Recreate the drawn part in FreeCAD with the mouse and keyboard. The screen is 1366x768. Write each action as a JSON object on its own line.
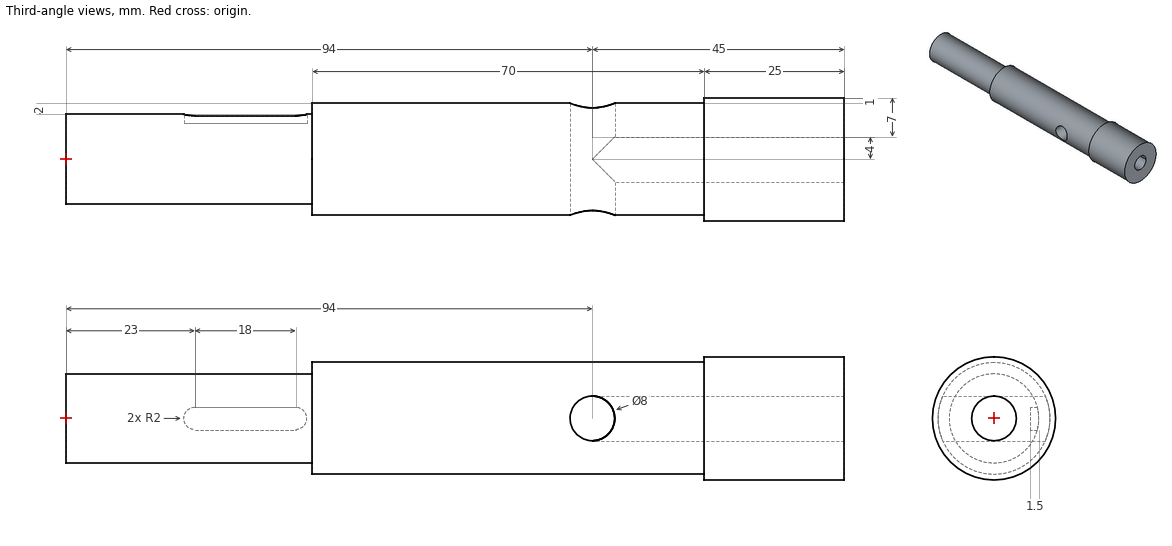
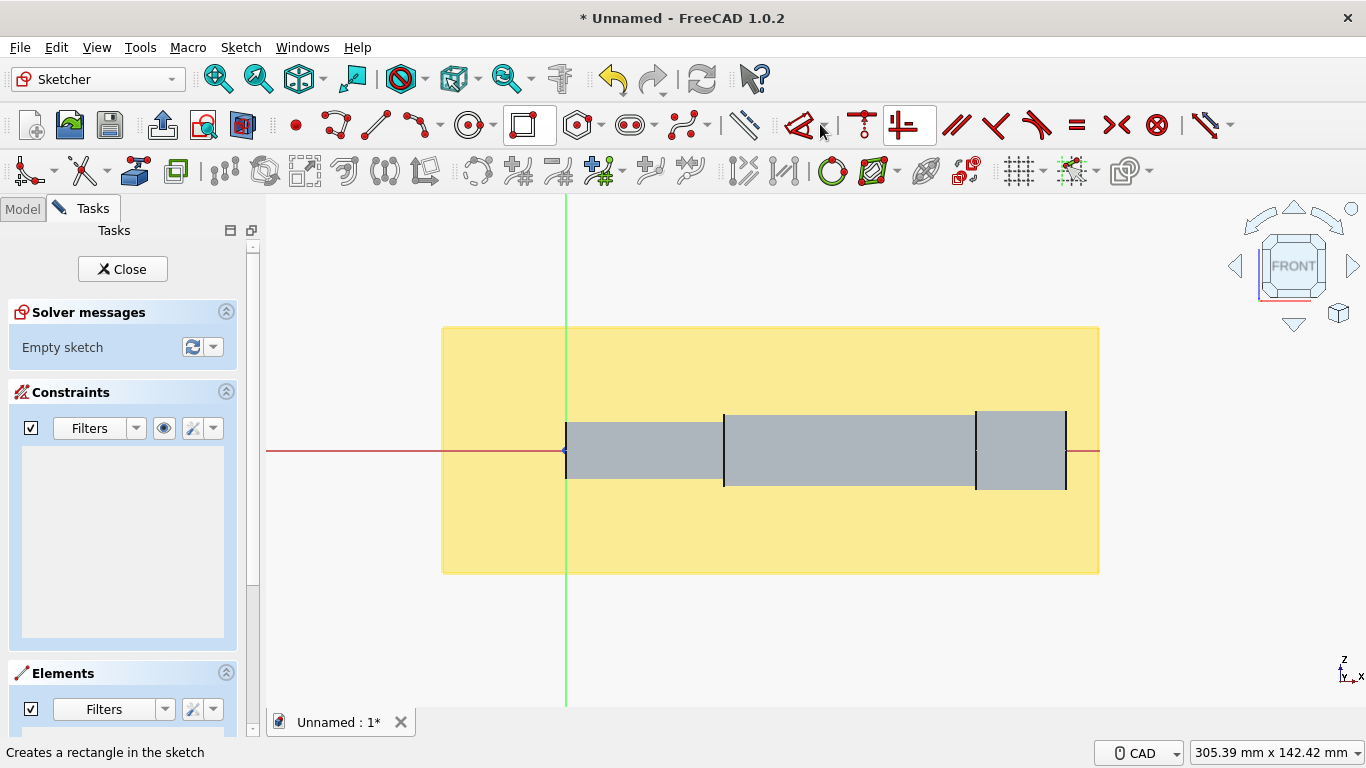
{"action": "key", "text": "q s"}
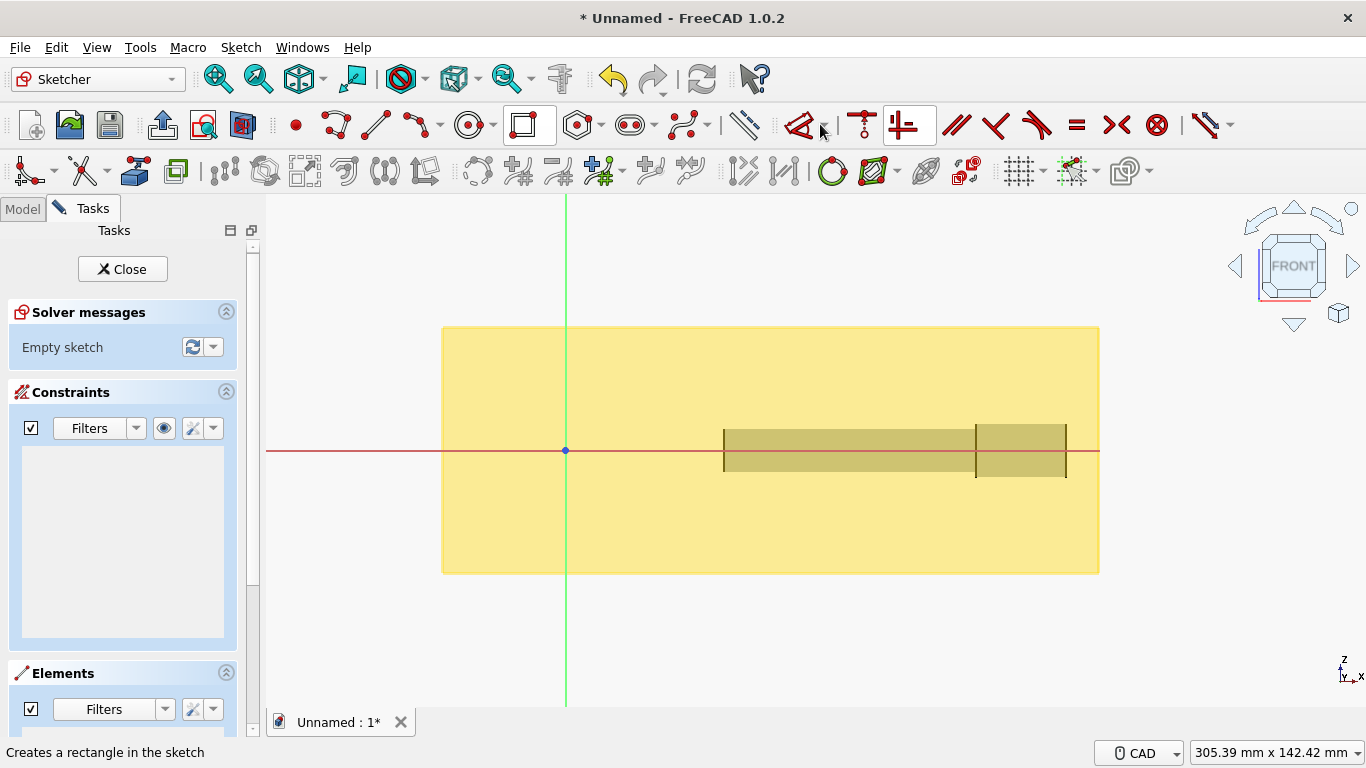
{"action": "scroll", "coordinate": [609, 450], "scroll_direction": "up", "scroll_amount": 7}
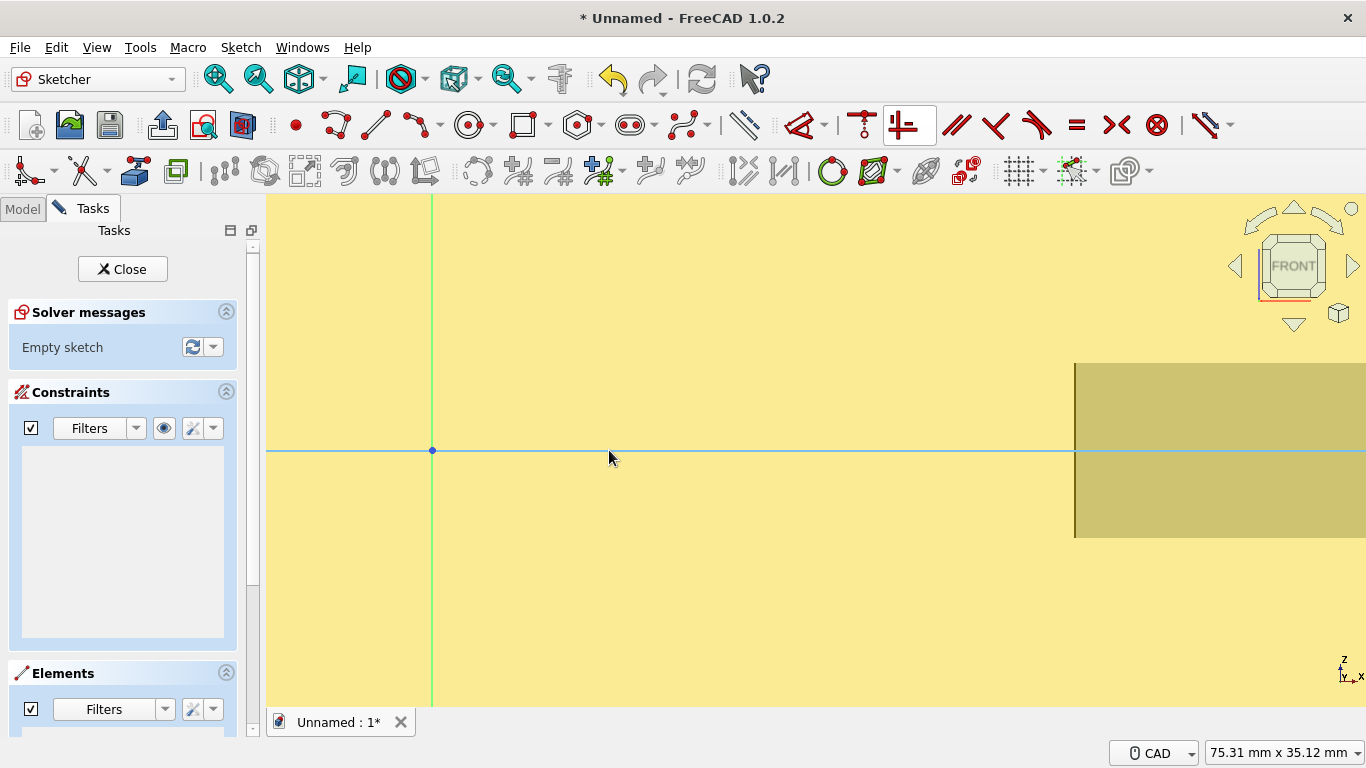
{"action": "left_click", "coordinate": [630, 126]}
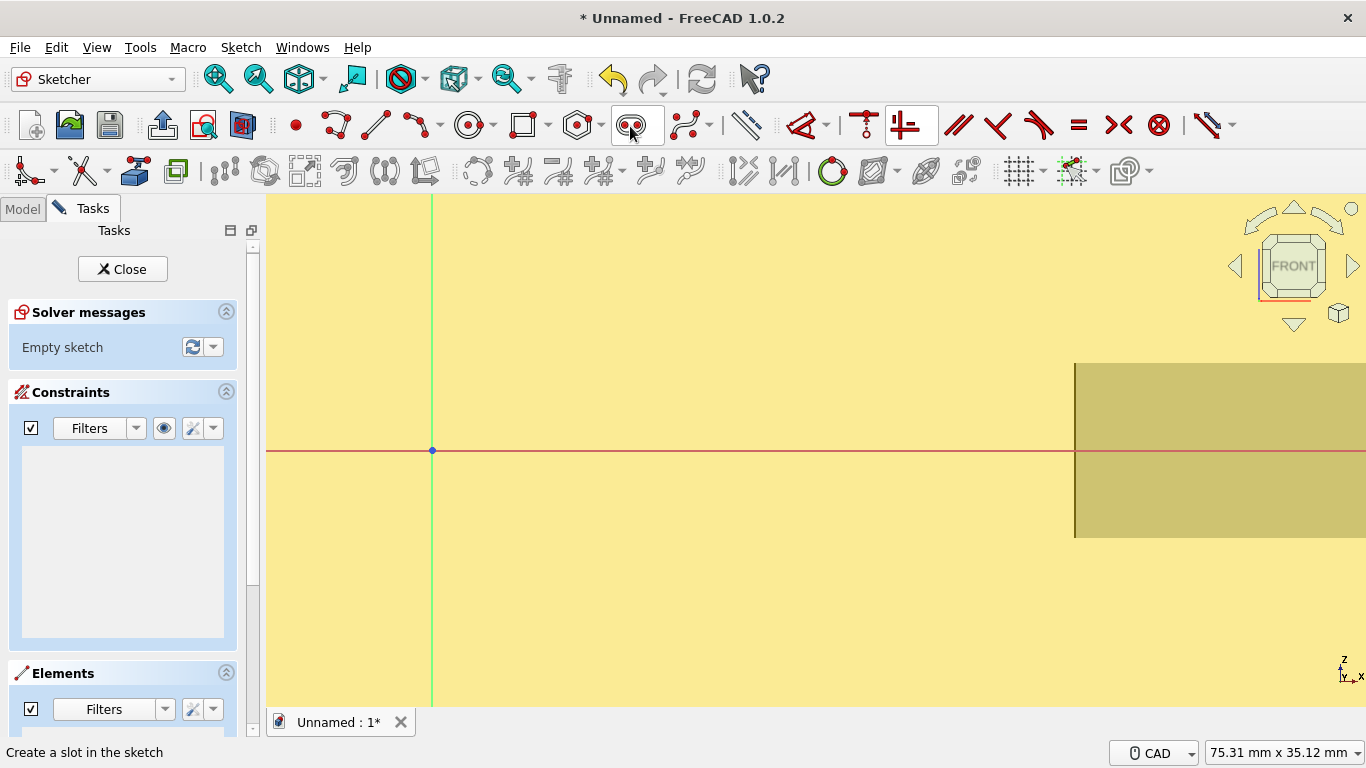
{"action": "left_click", "coordinate": [768, 450]}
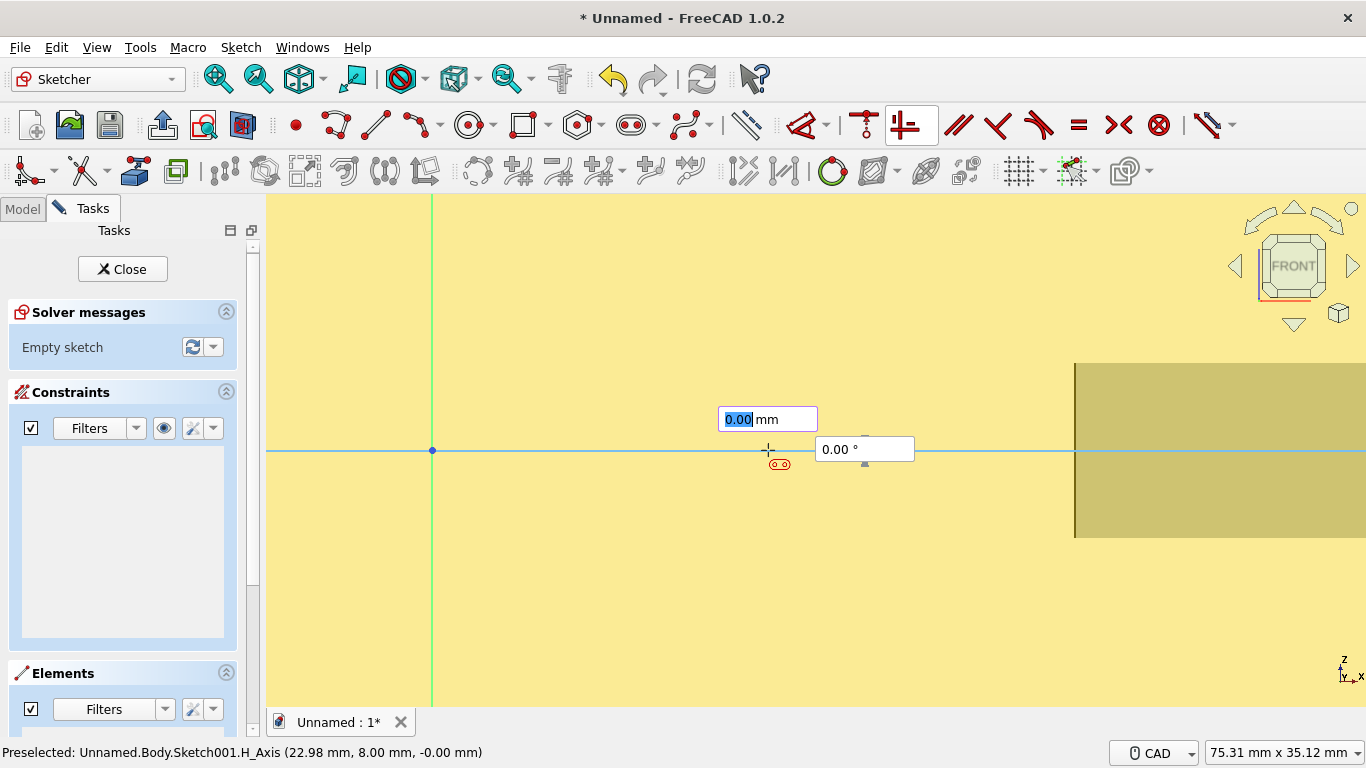
{"action": "left_click", "coordinate": [1031, 442]}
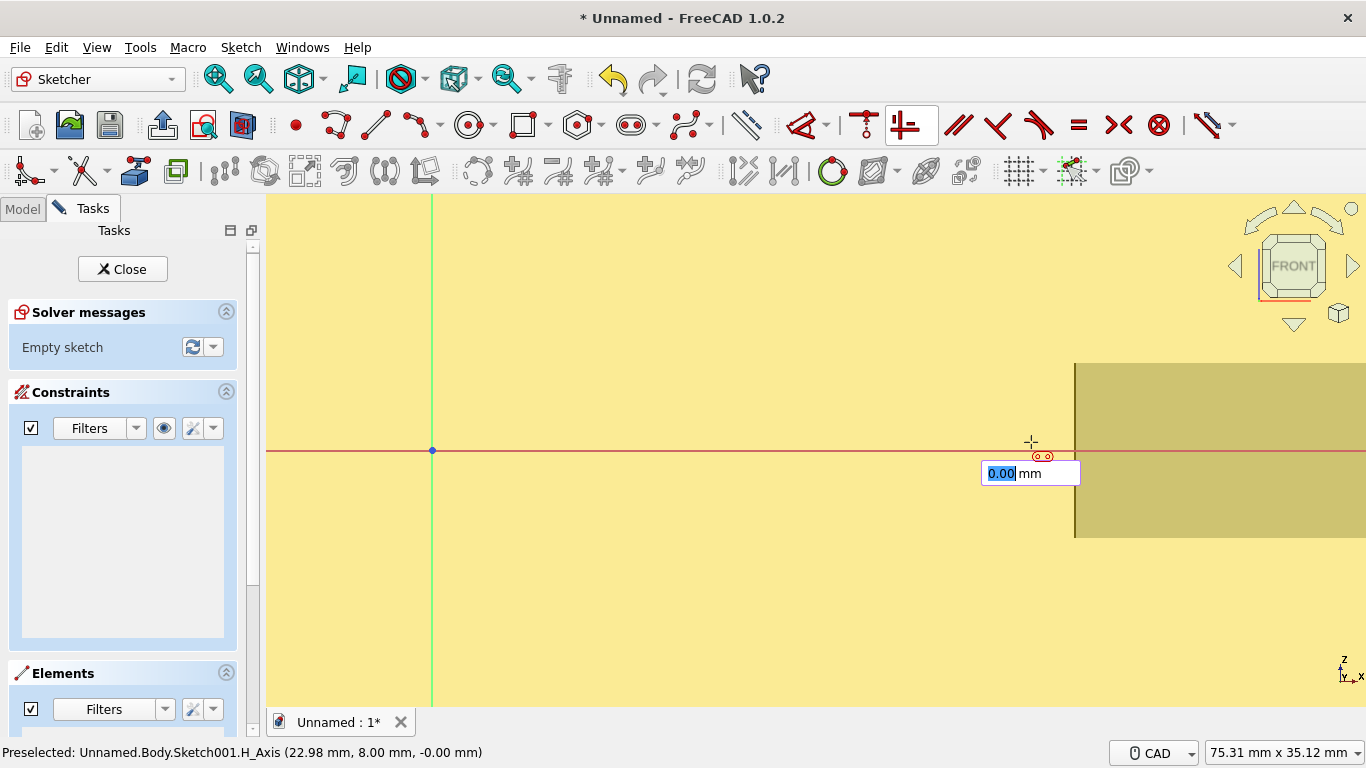
{"action": "left_click", "coordinate": [900, 480]}
{"action": "key", "text": "Escape"}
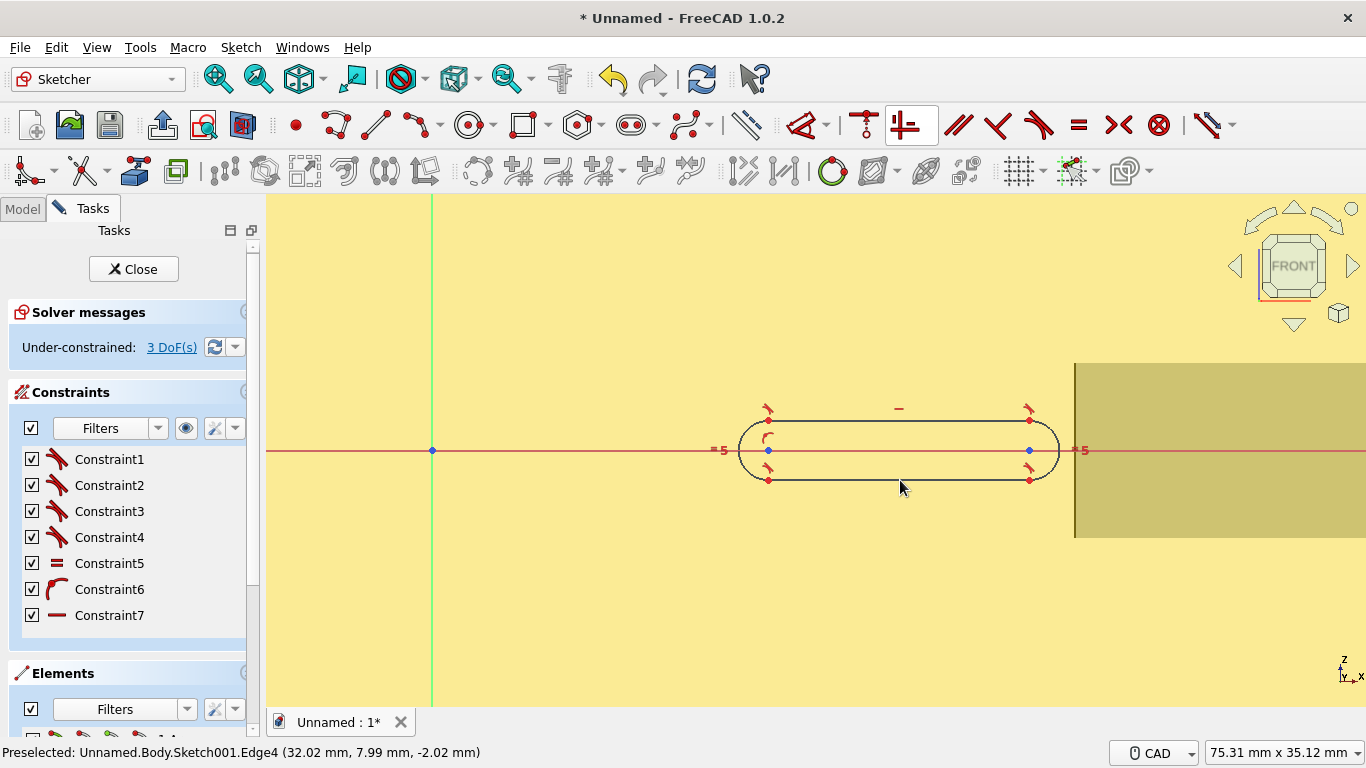
{"action": "key", "text": "d"}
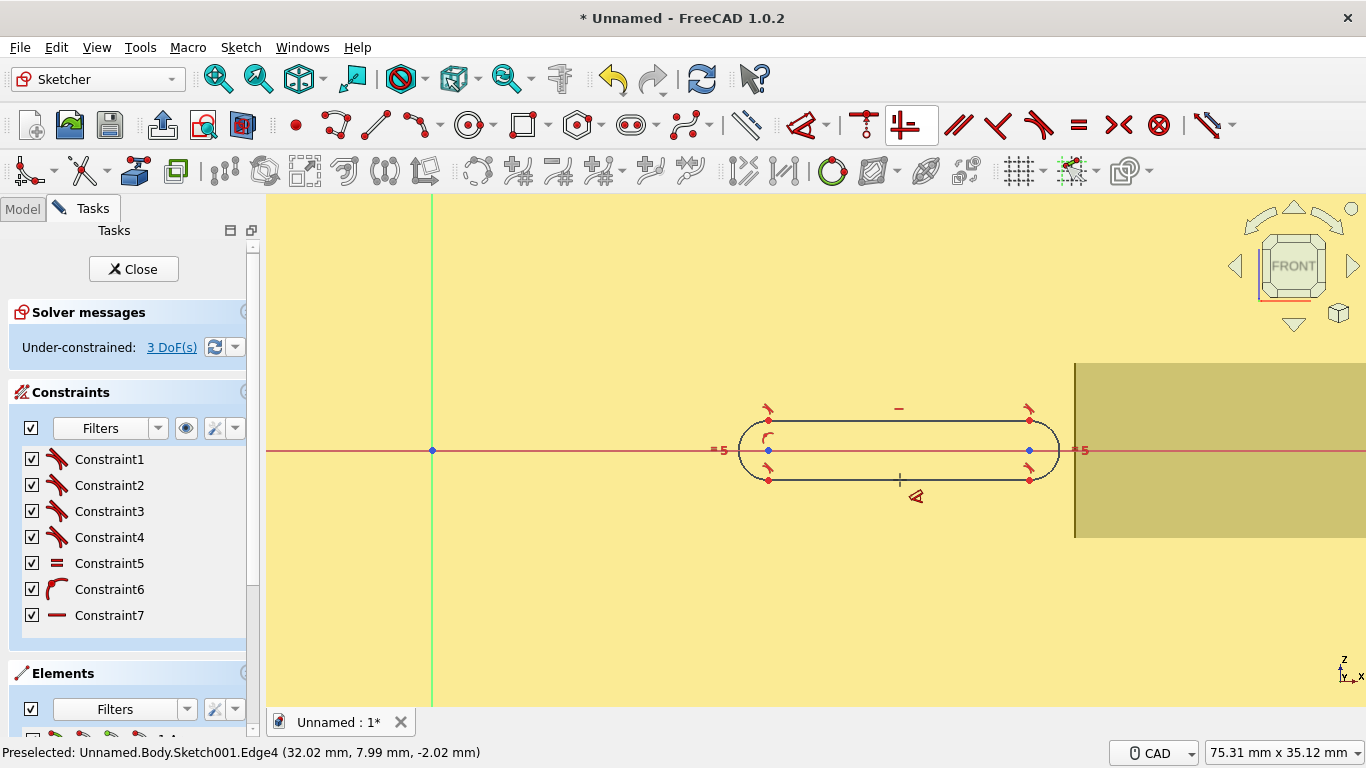
{"action": "scroll", "coordinate": [745, 433], "scroll_direction": "up", "scroll_amount": 2}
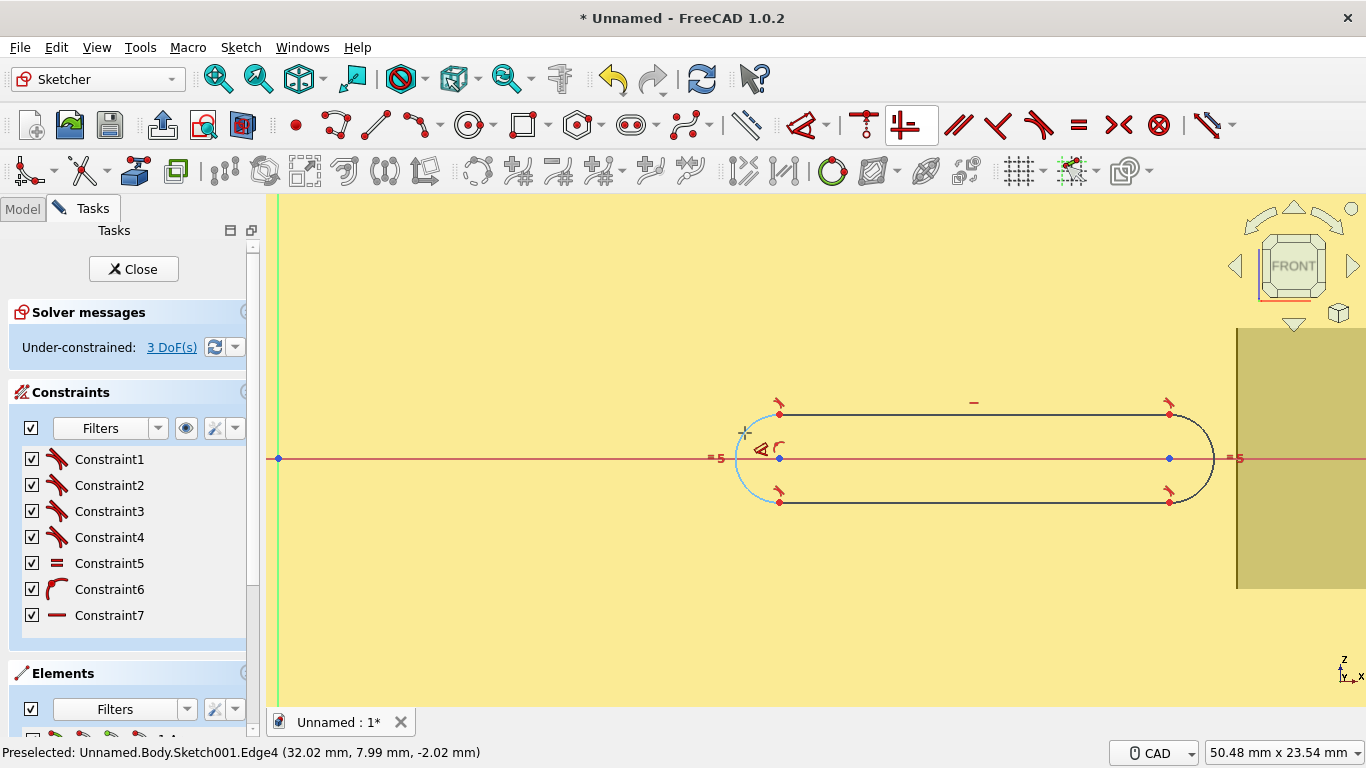
{"action": "left_click", "coordinate": [744, 433]}
{"action": "left_click", "coordinate": [718, 414]}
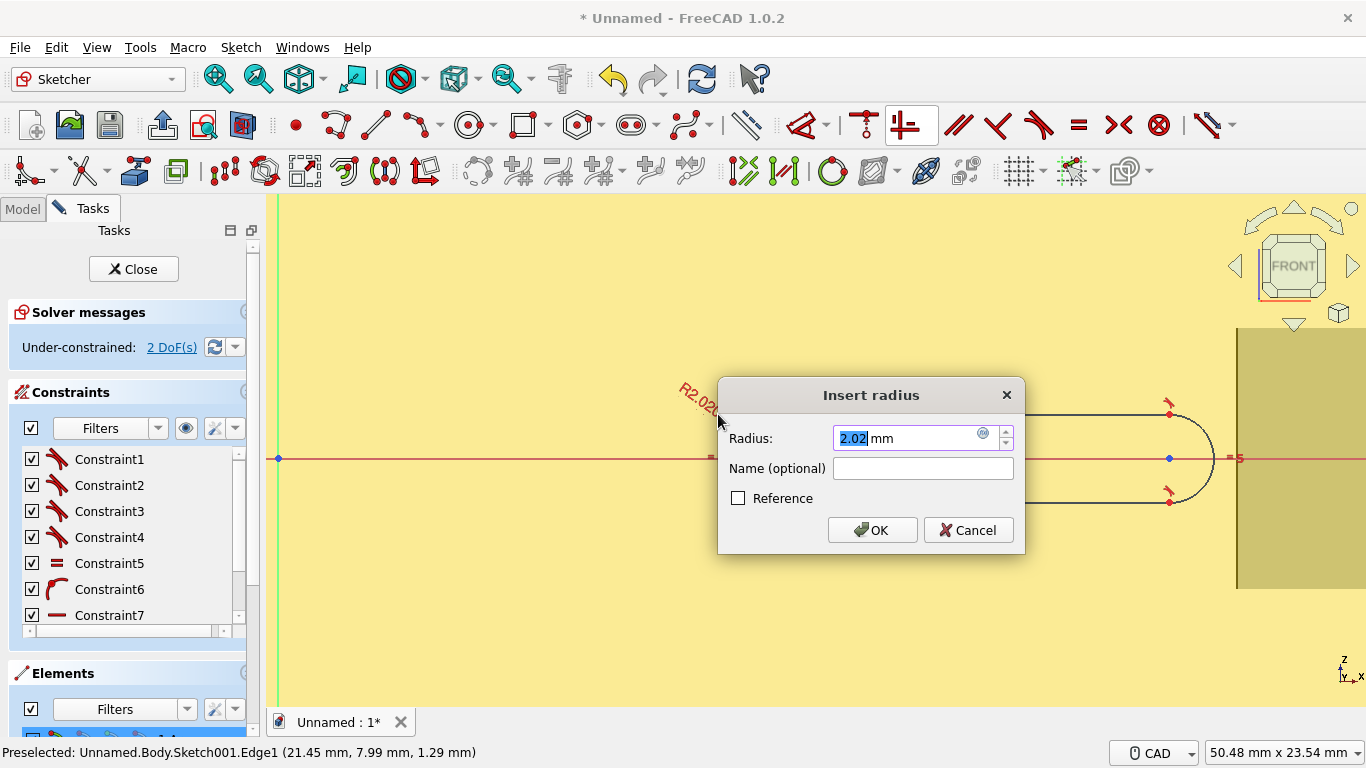
{"action": "type", "text": "2"}
{"action": "key", "text": "Return"}